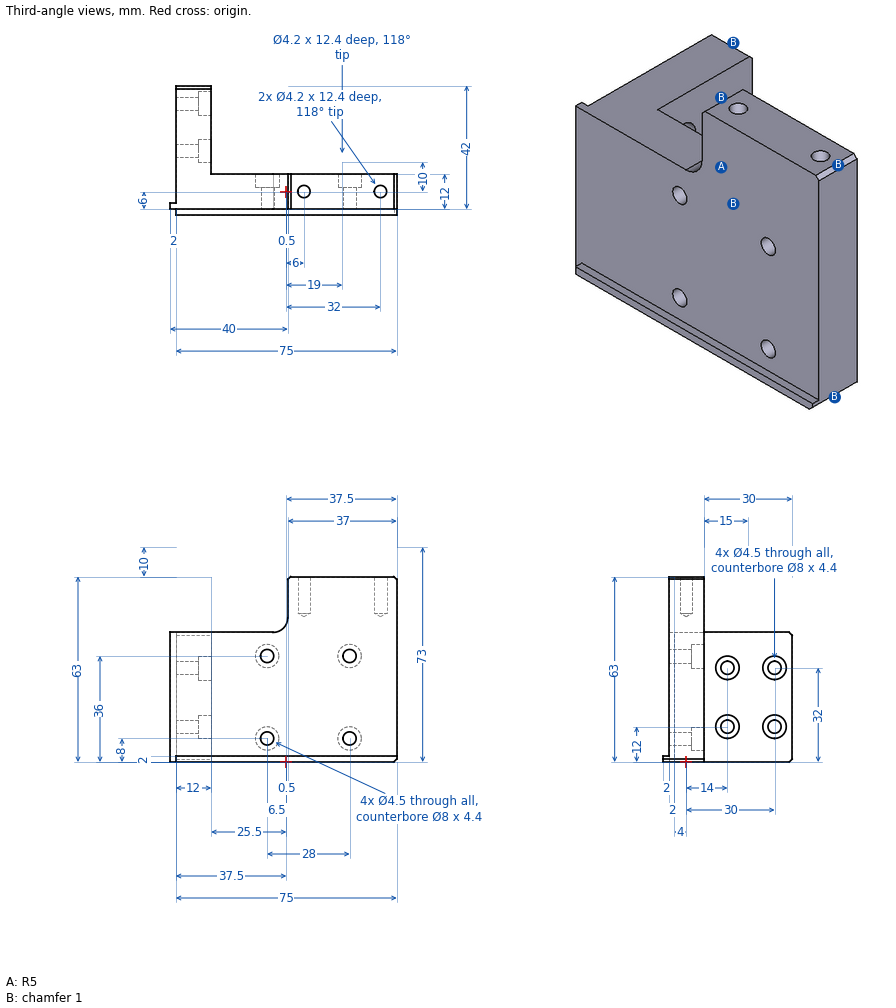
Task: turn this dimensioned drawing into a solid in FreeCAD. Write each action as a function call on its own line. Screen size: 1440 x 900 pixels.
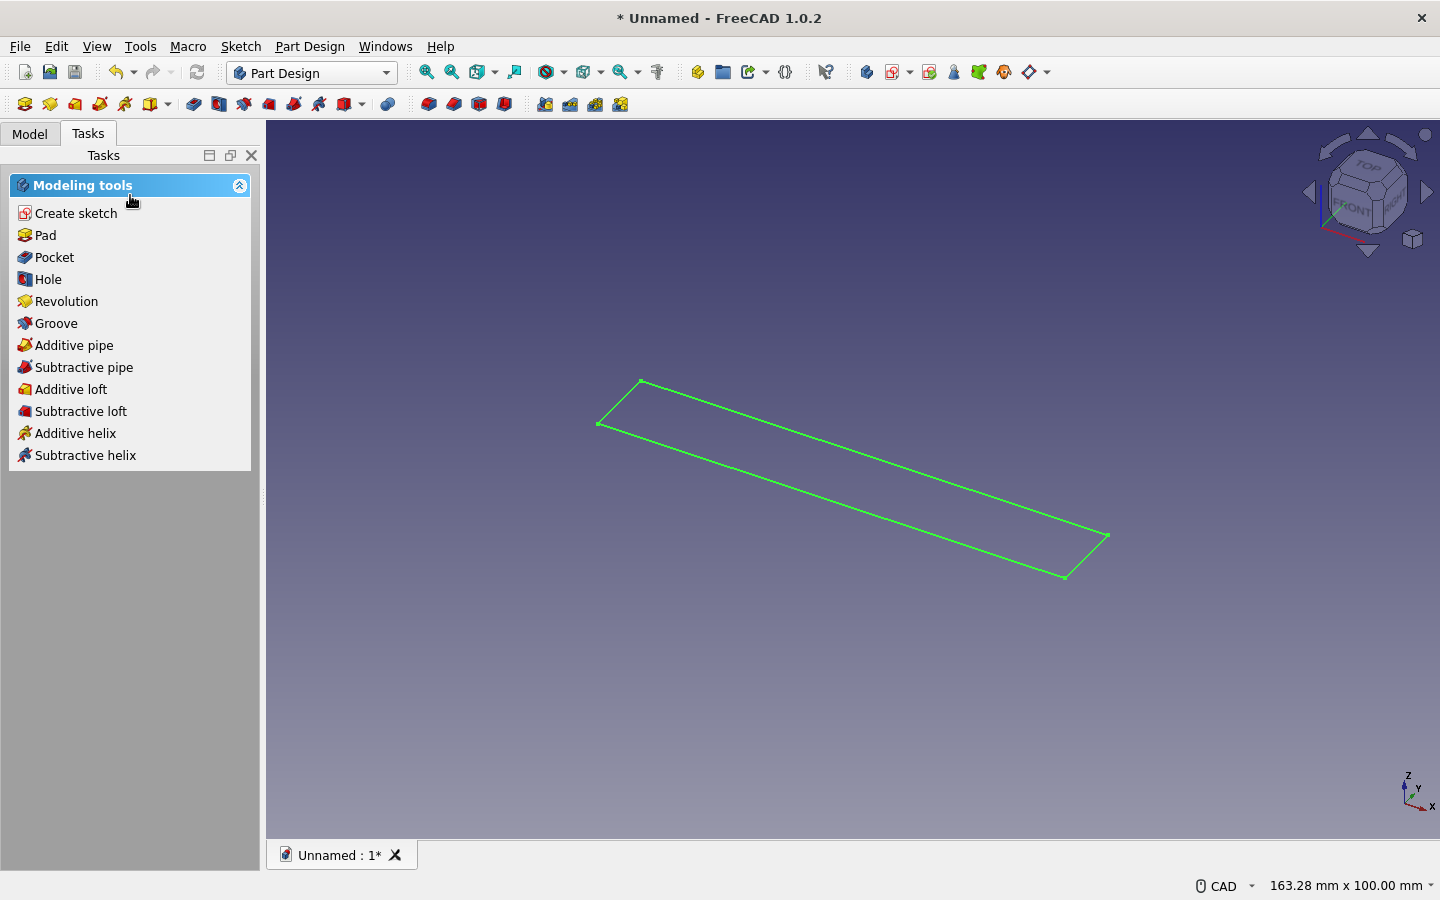
click(25, 104)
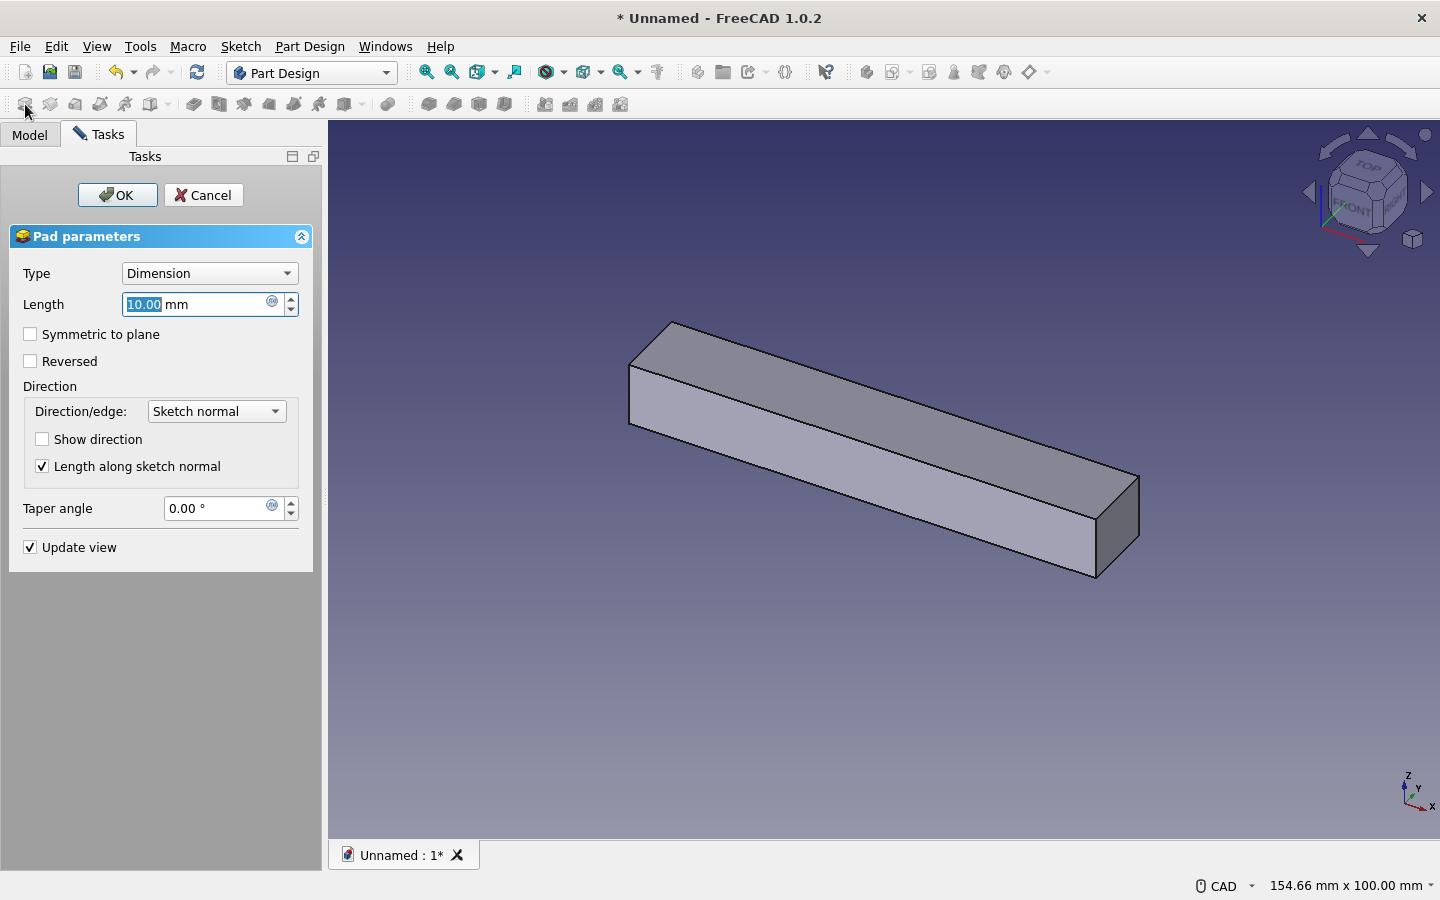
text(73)
key(Tab)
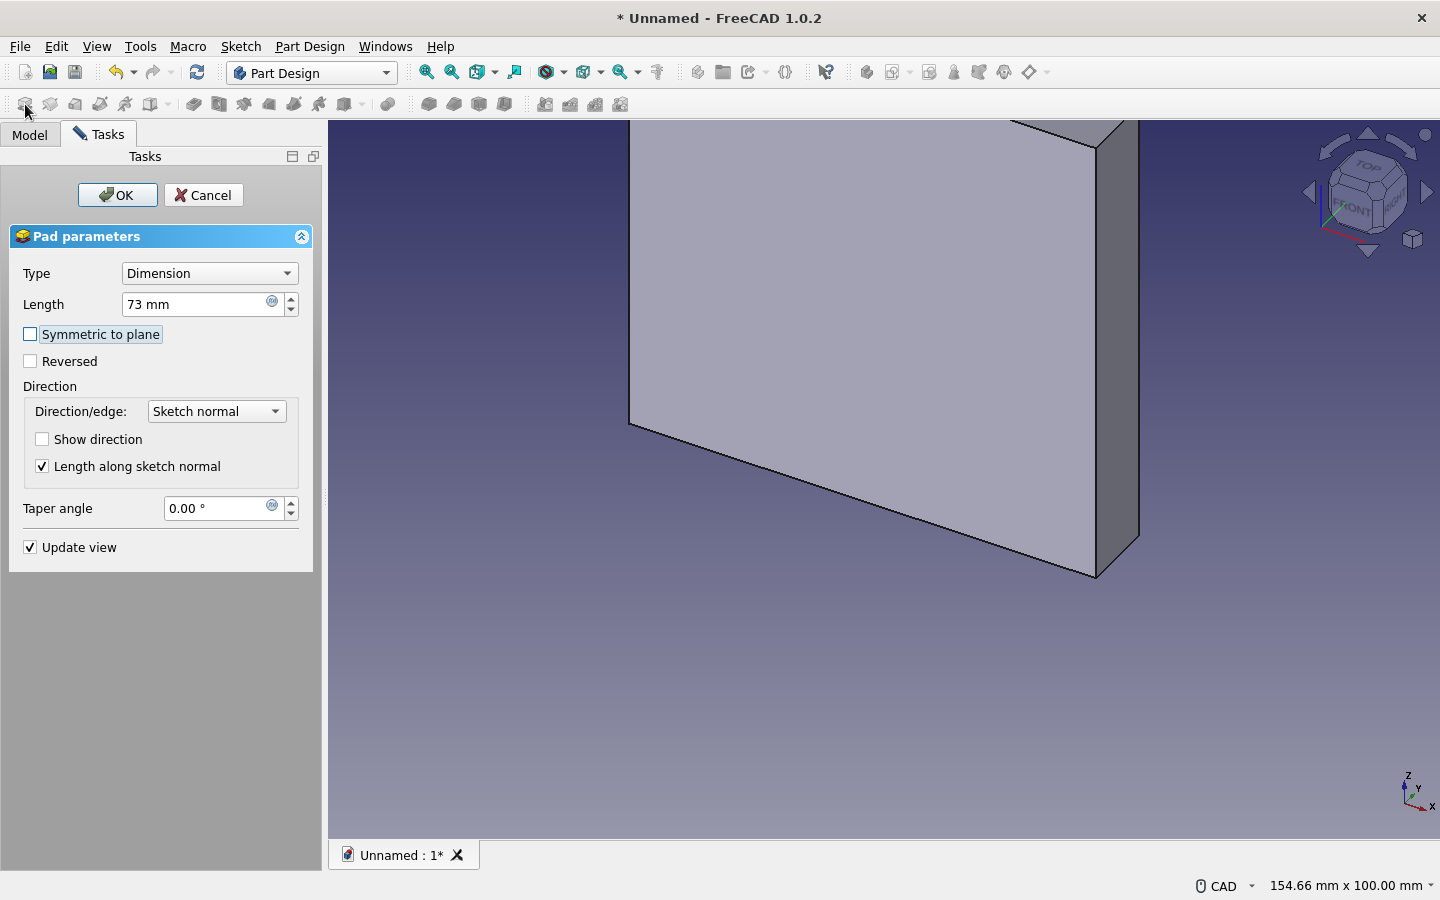
click(118, 195)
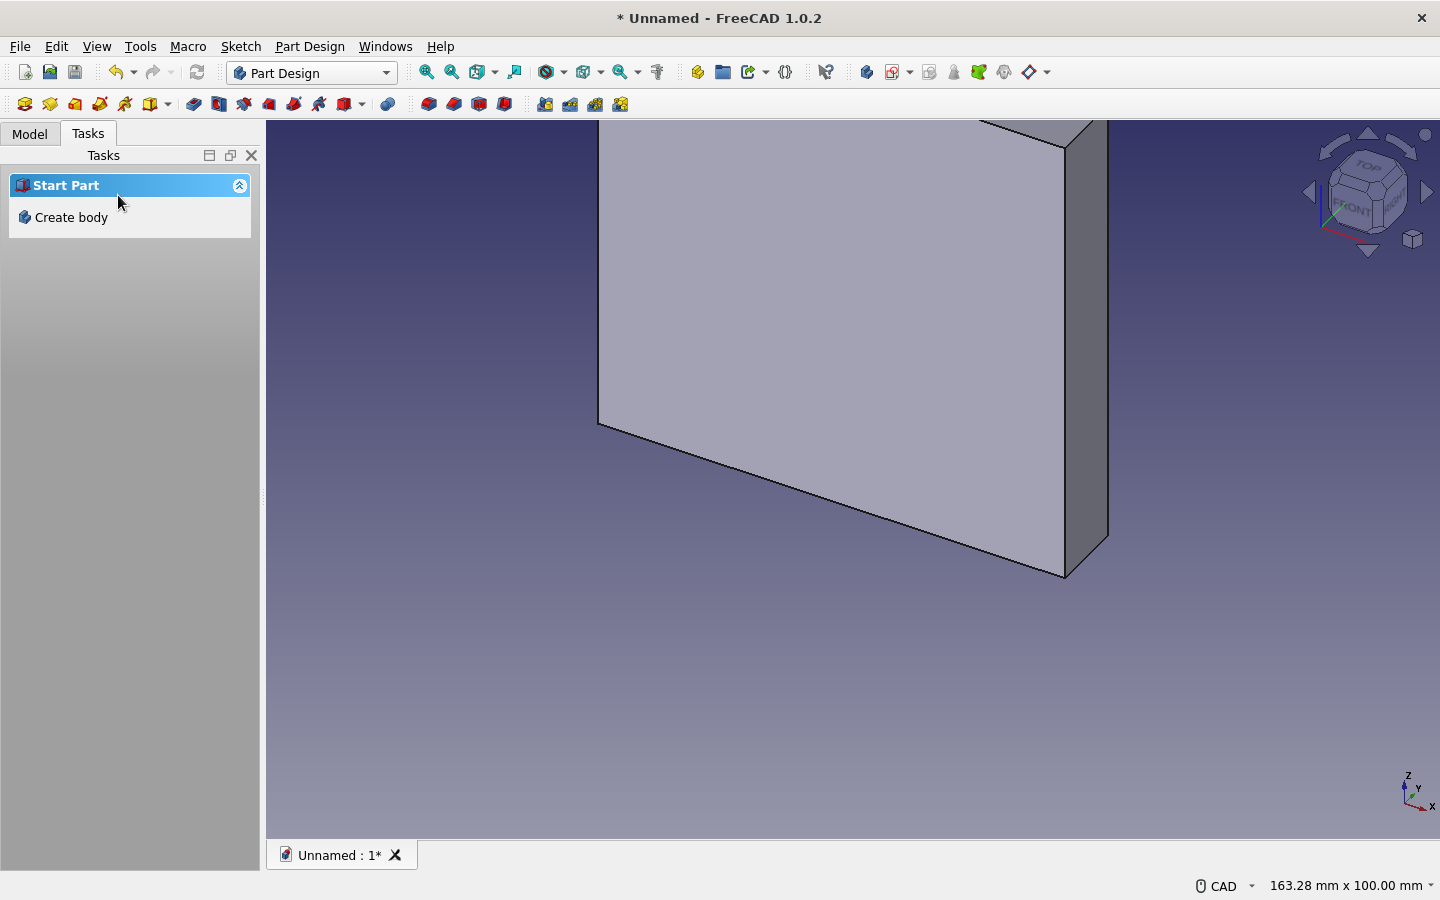
click(427, 72)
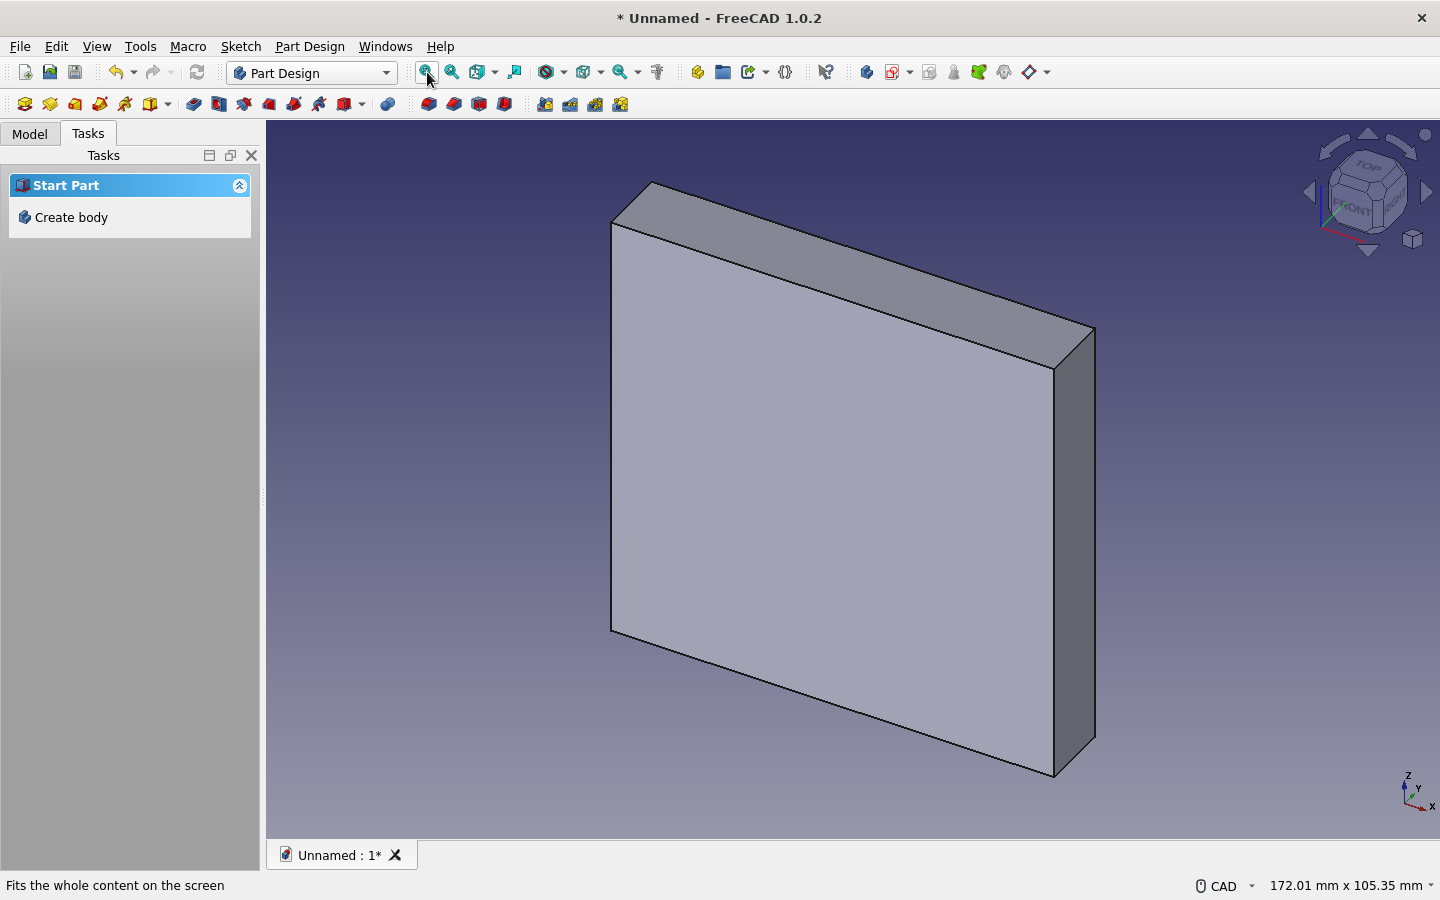
click(833, 499)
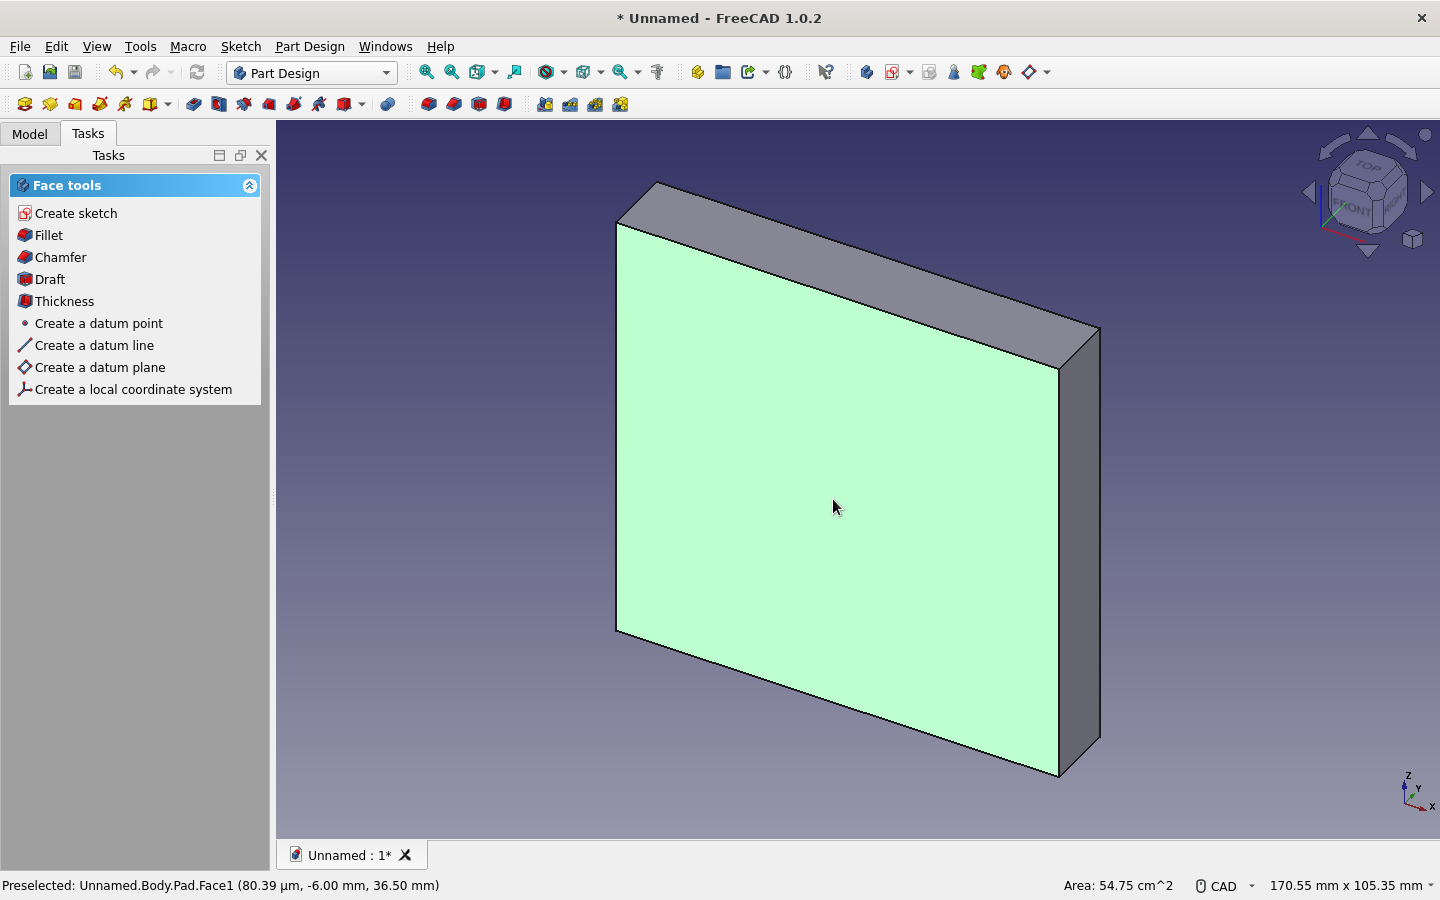
click(892, 72)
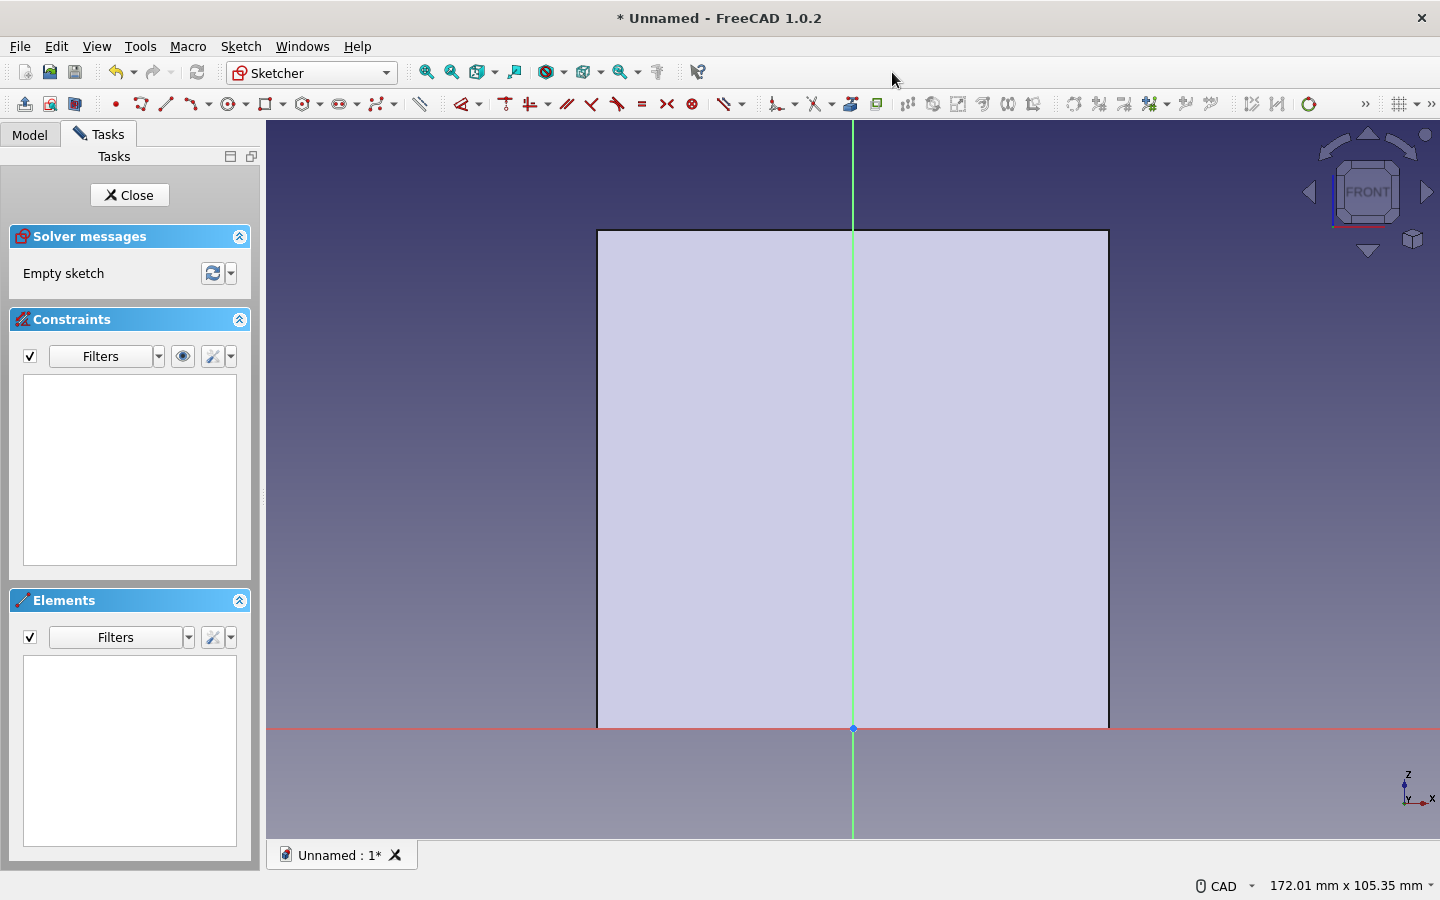
scroll(992, 811, up, 2)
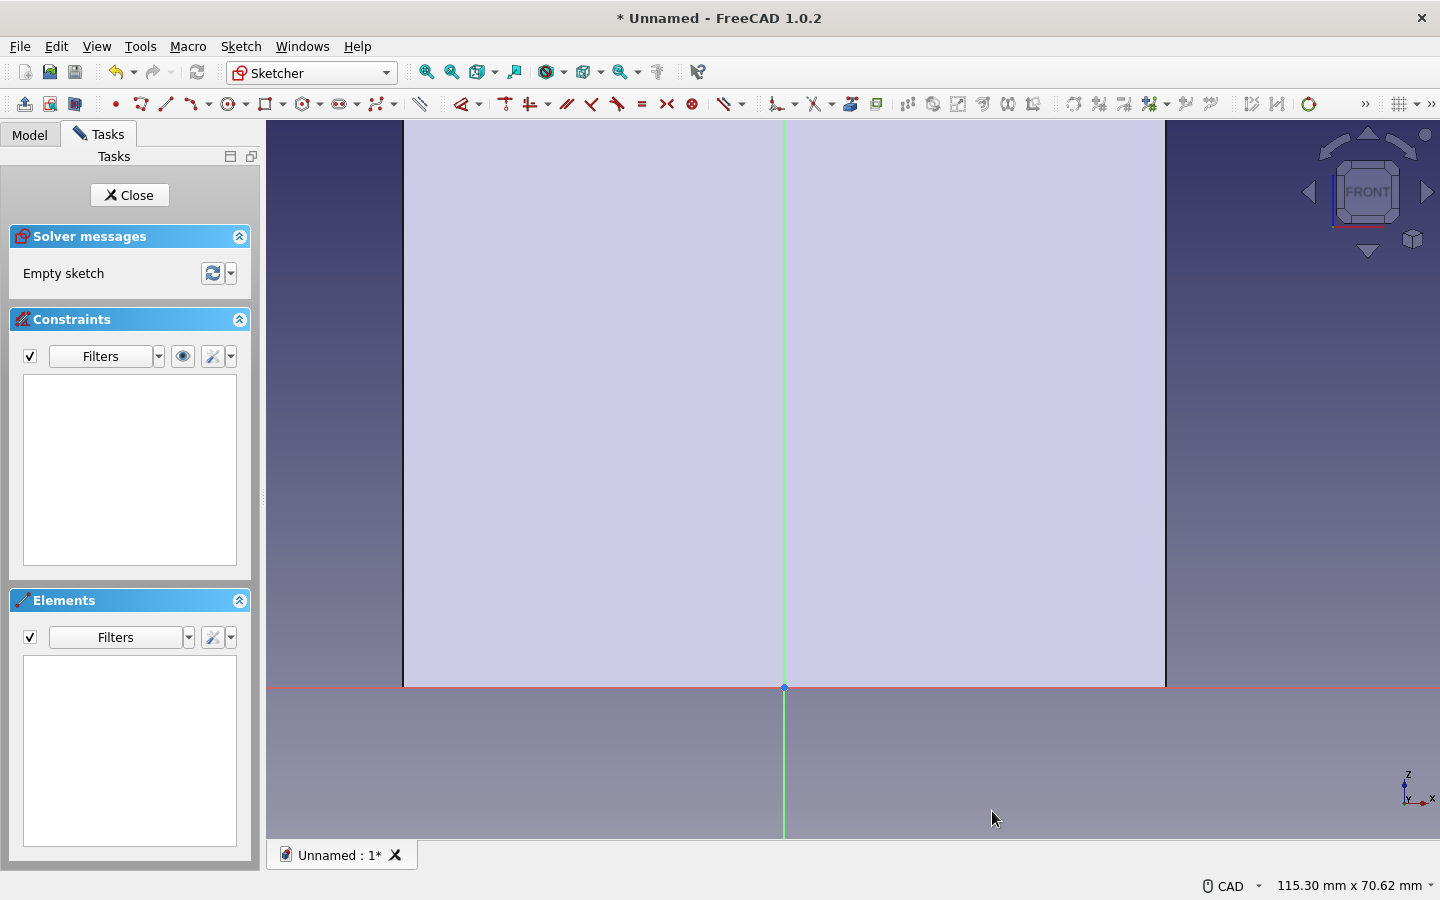
click(264, 104)